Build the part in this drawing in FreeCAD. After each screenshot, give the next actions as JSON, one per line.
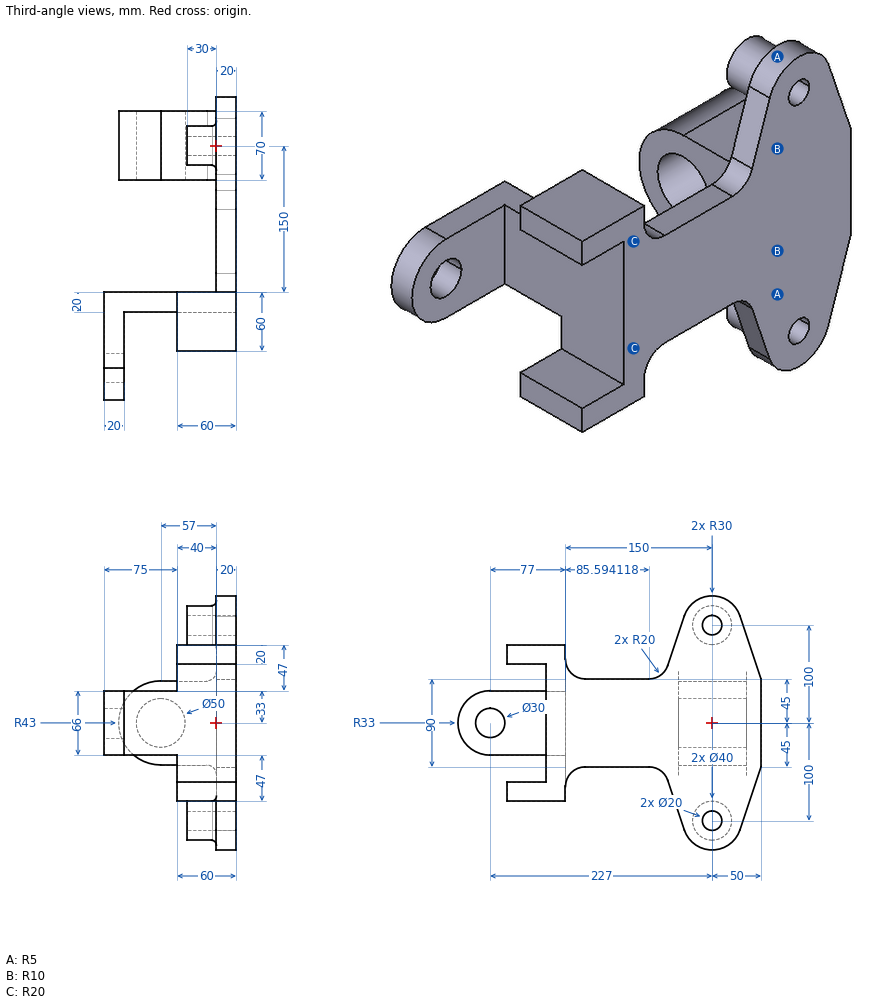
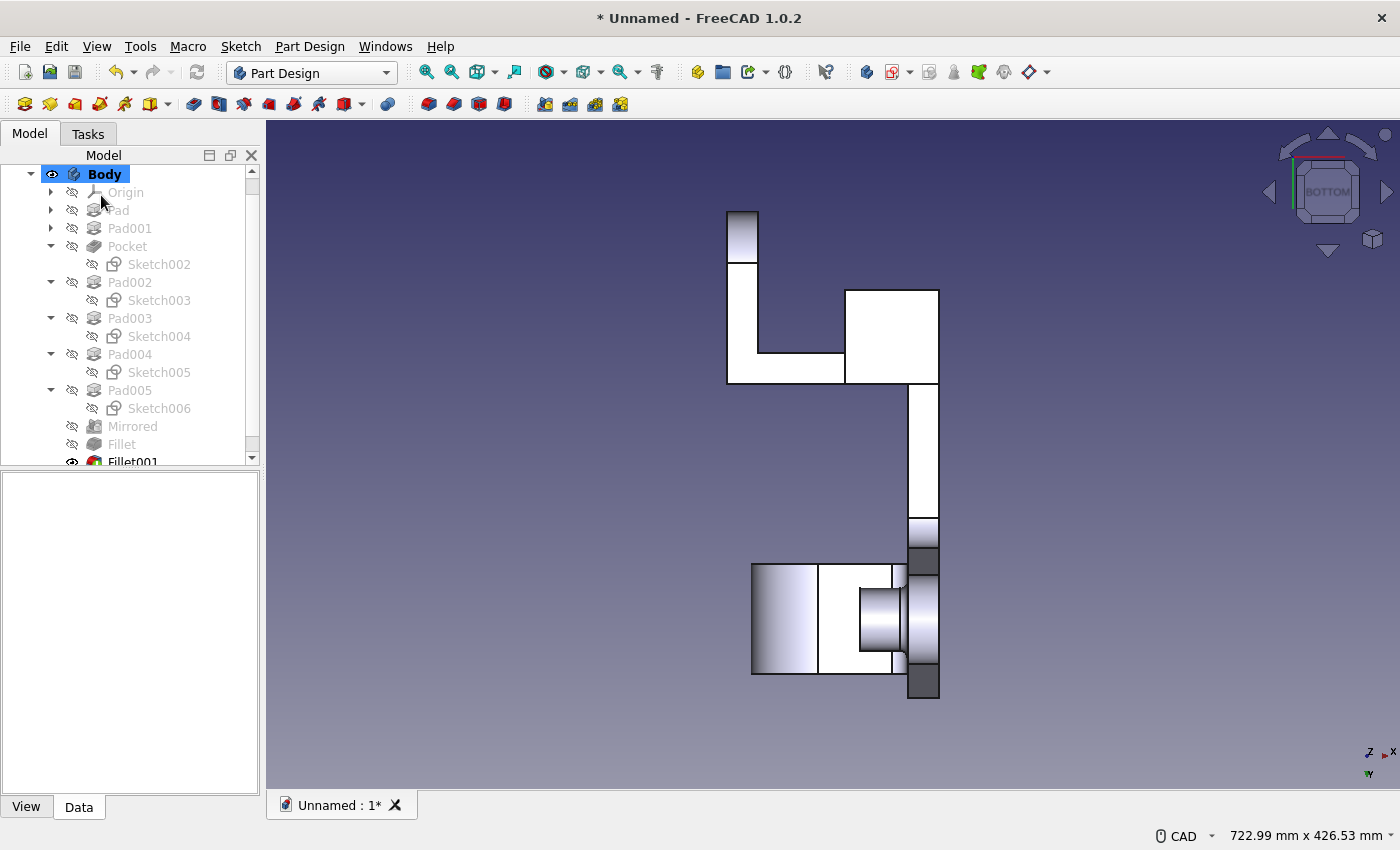
{"action": "key", "text": "4"}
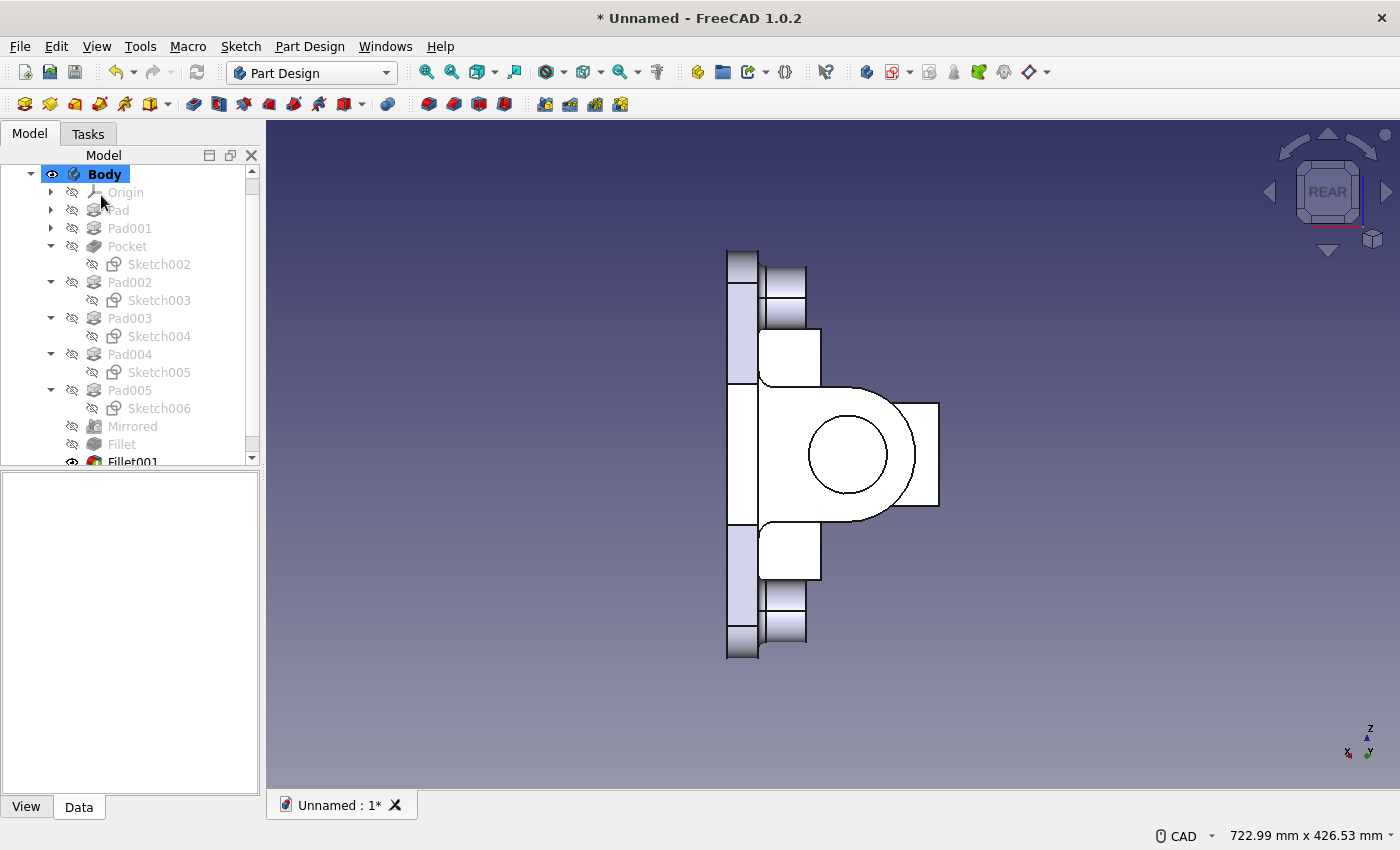
{"action": "key", "text": "6"}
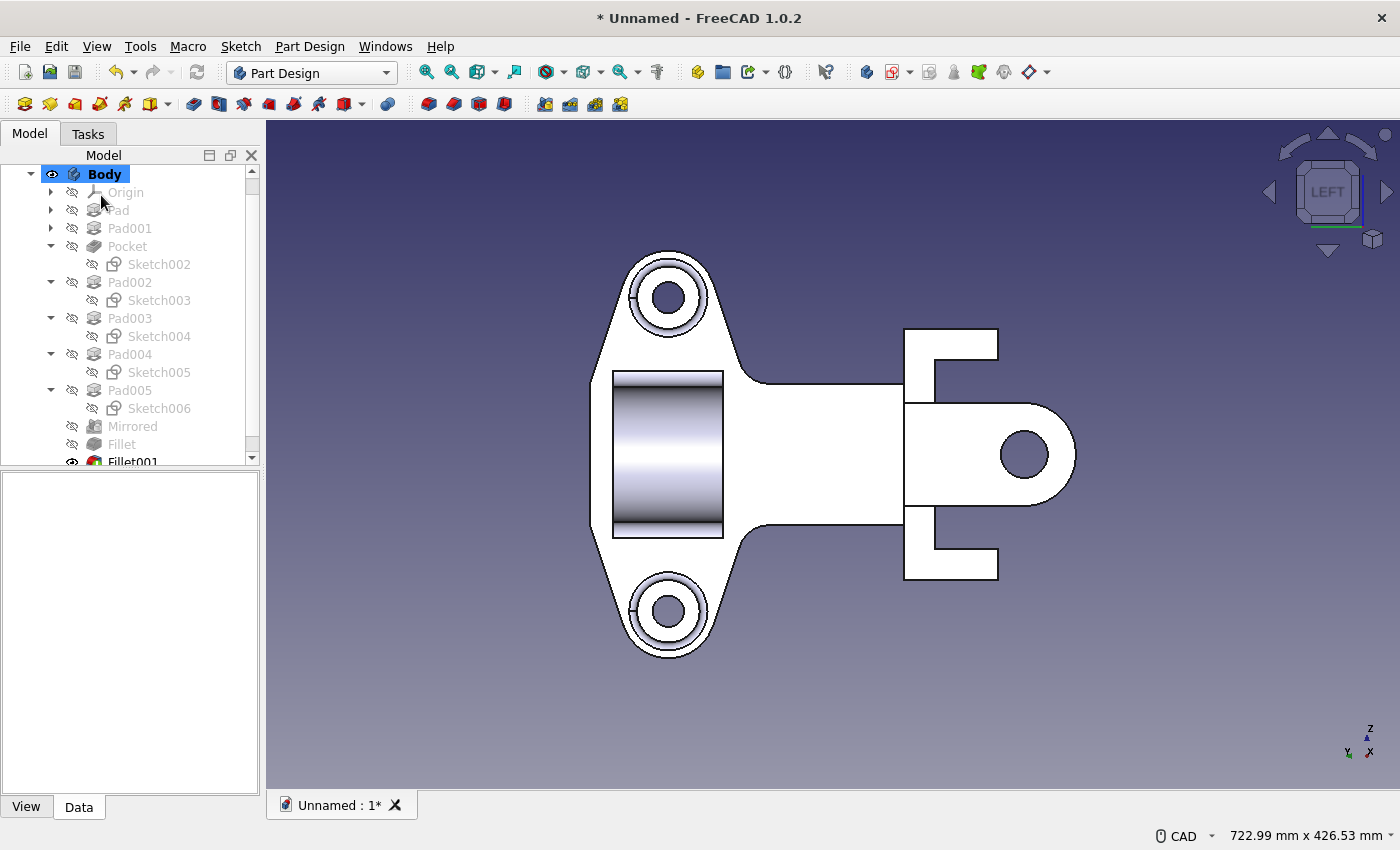
{"action": "key", "text": "v 3"}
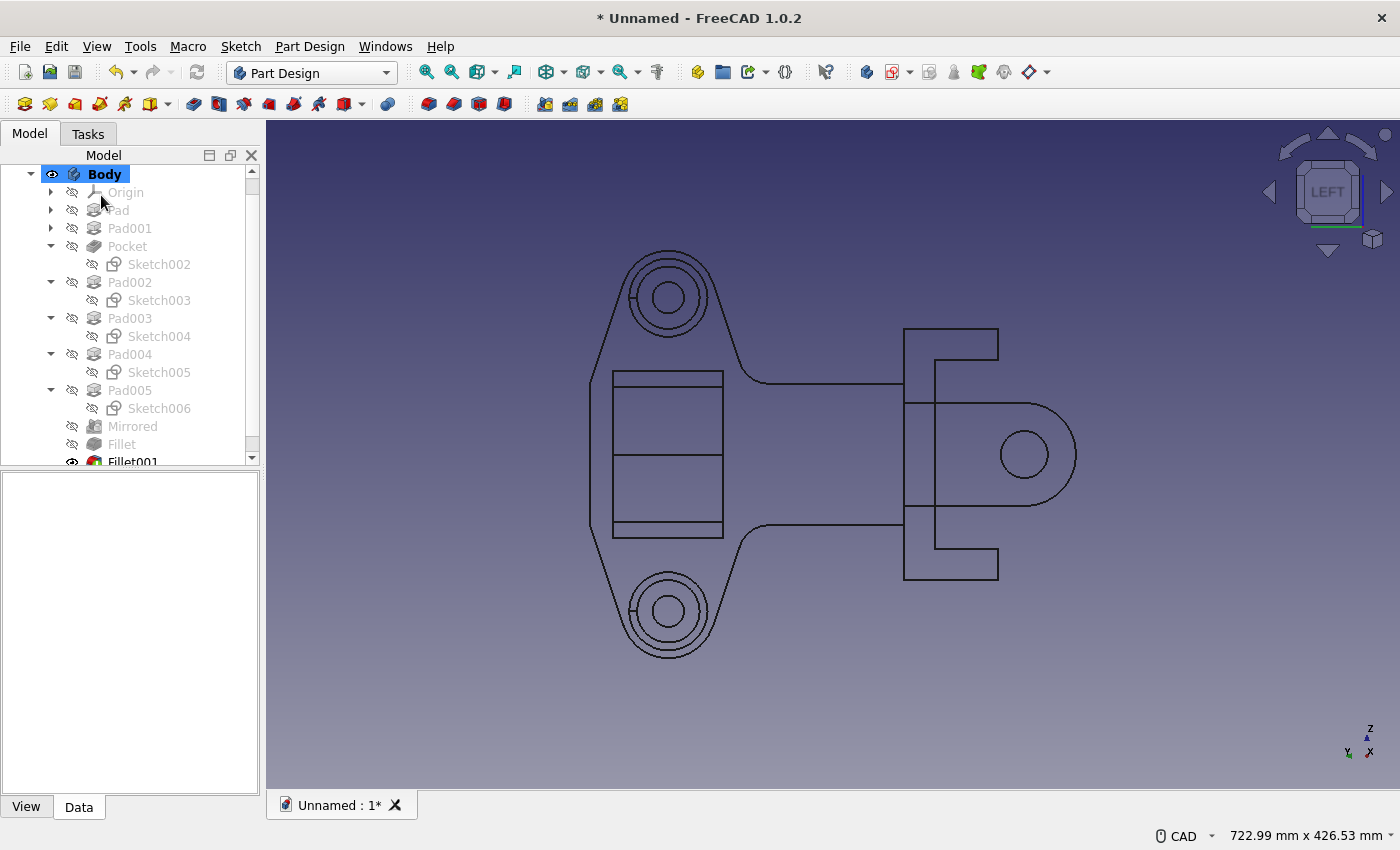
{"action": "key", "text": "0"}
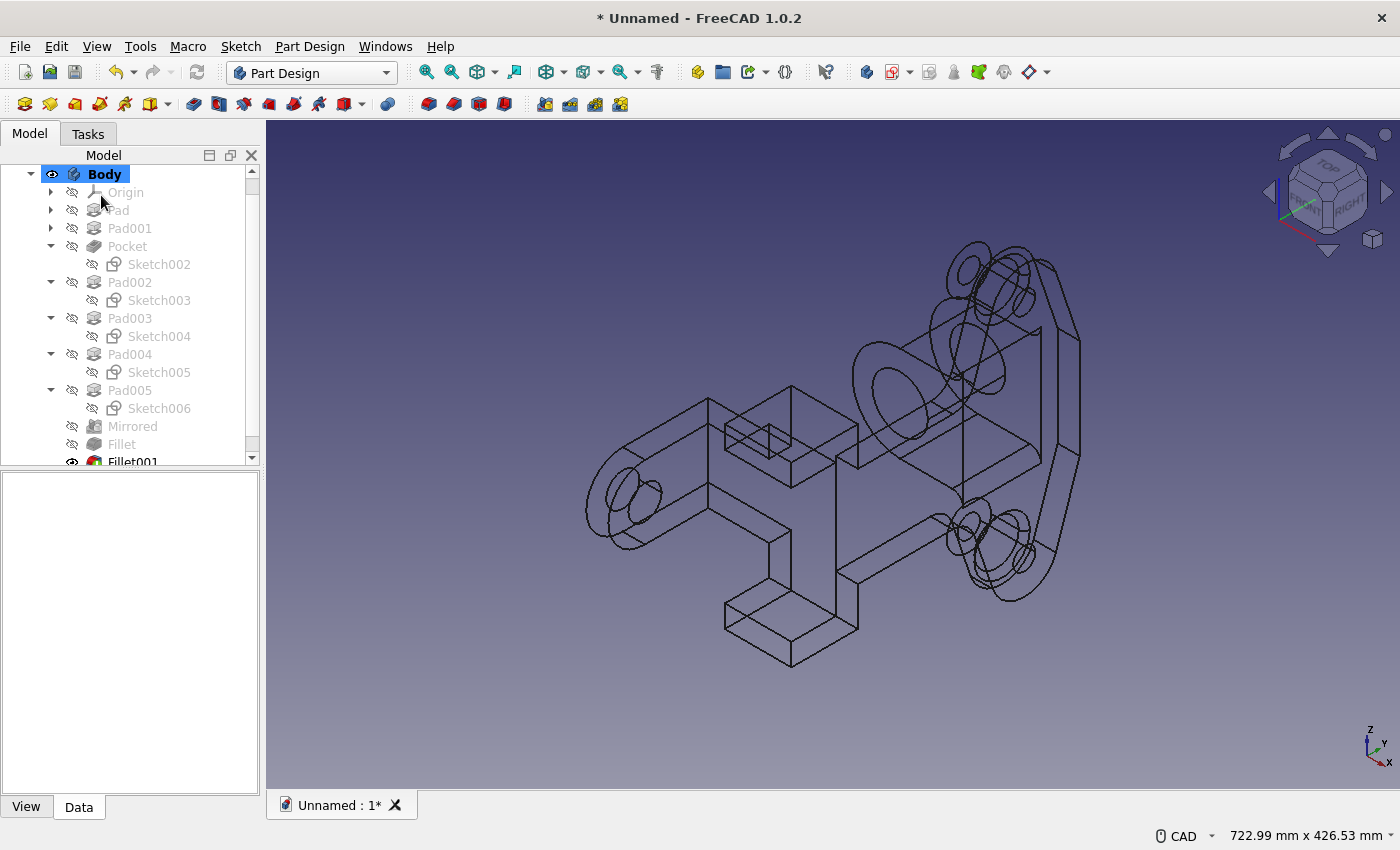
{"action": "left_click", "coordinate": [847, 577]}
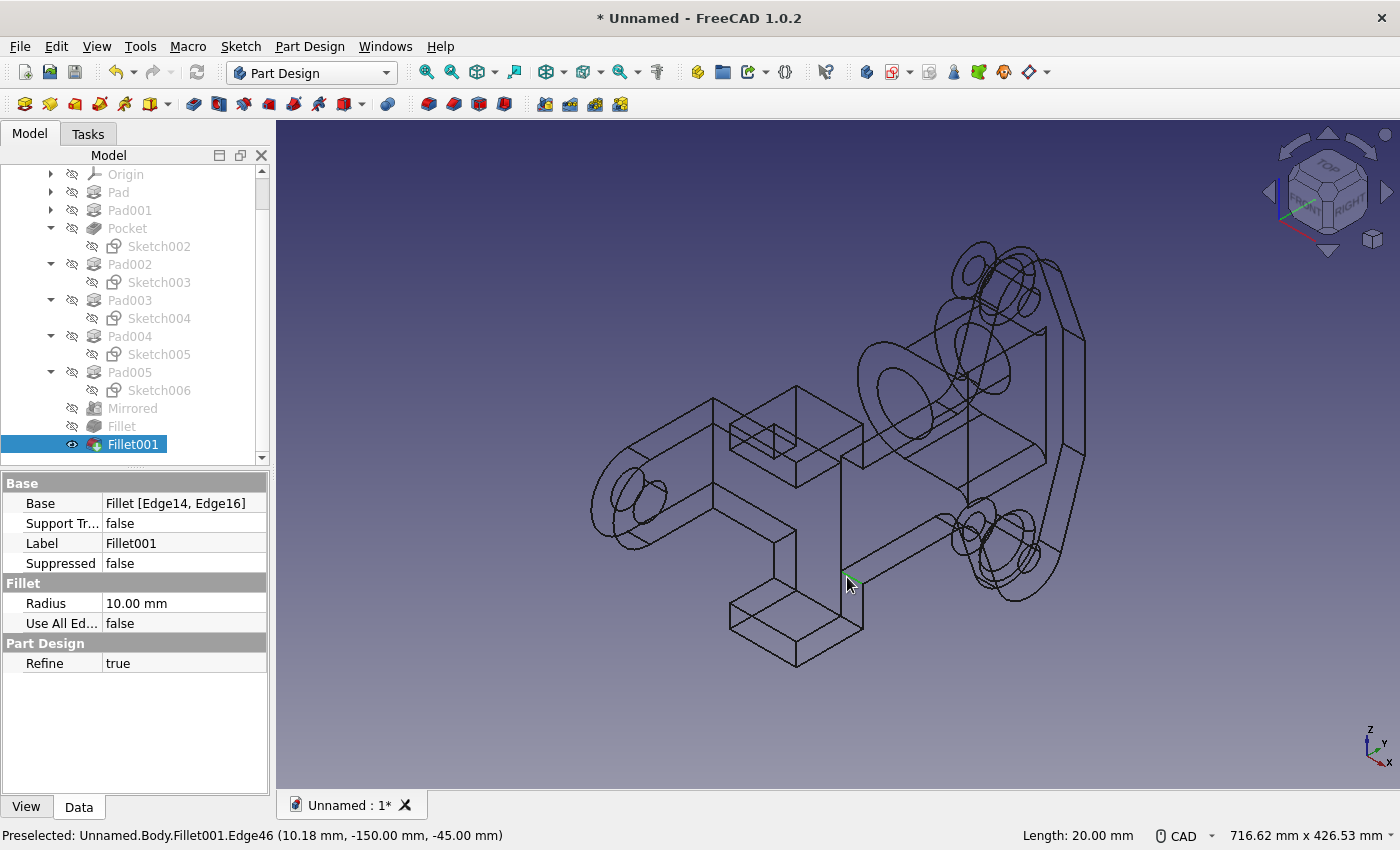
{"action": "left_click", "coordinate": [852, 462], "text": "ctrl"}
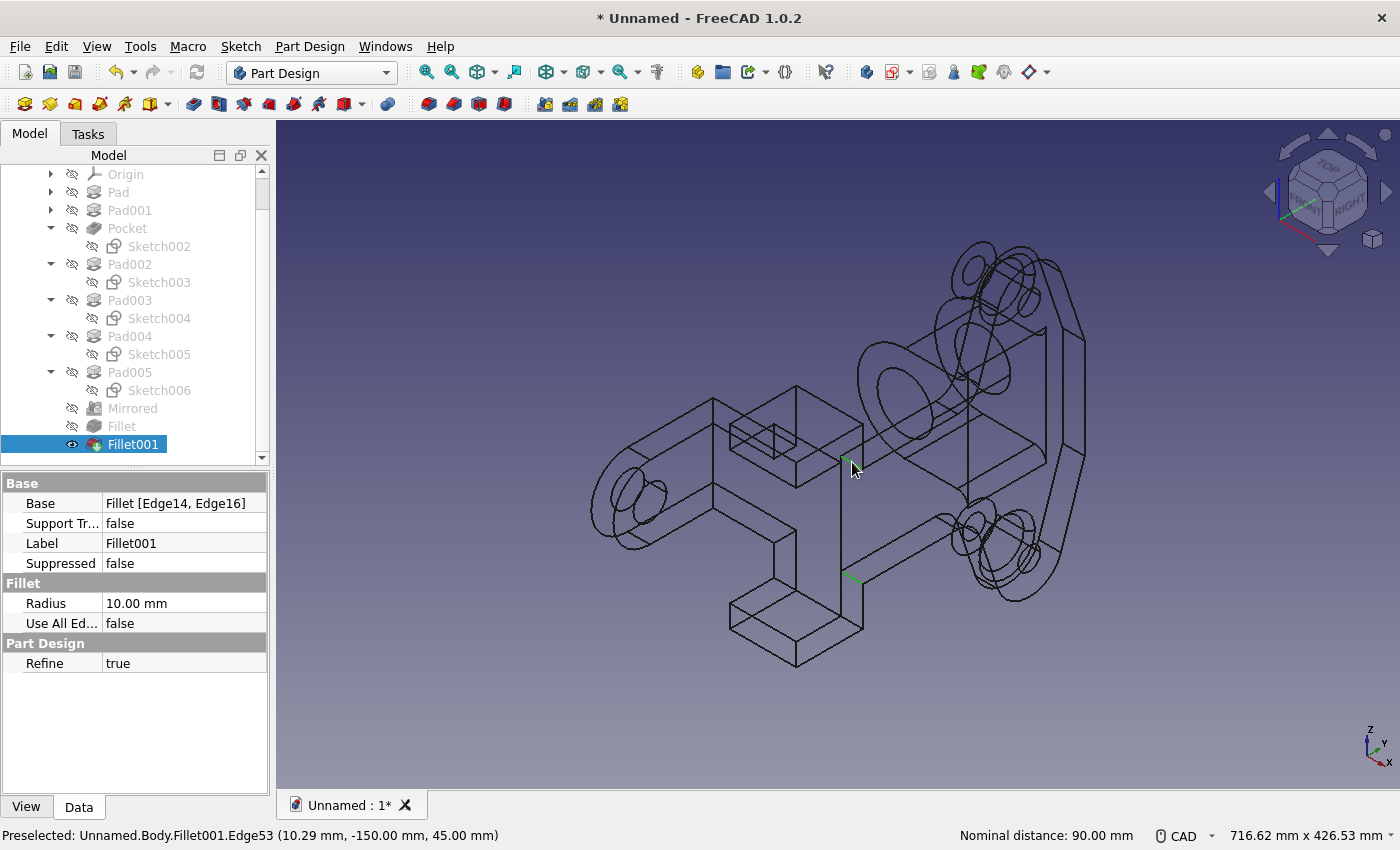
{"action": "key", "text": "v 1"}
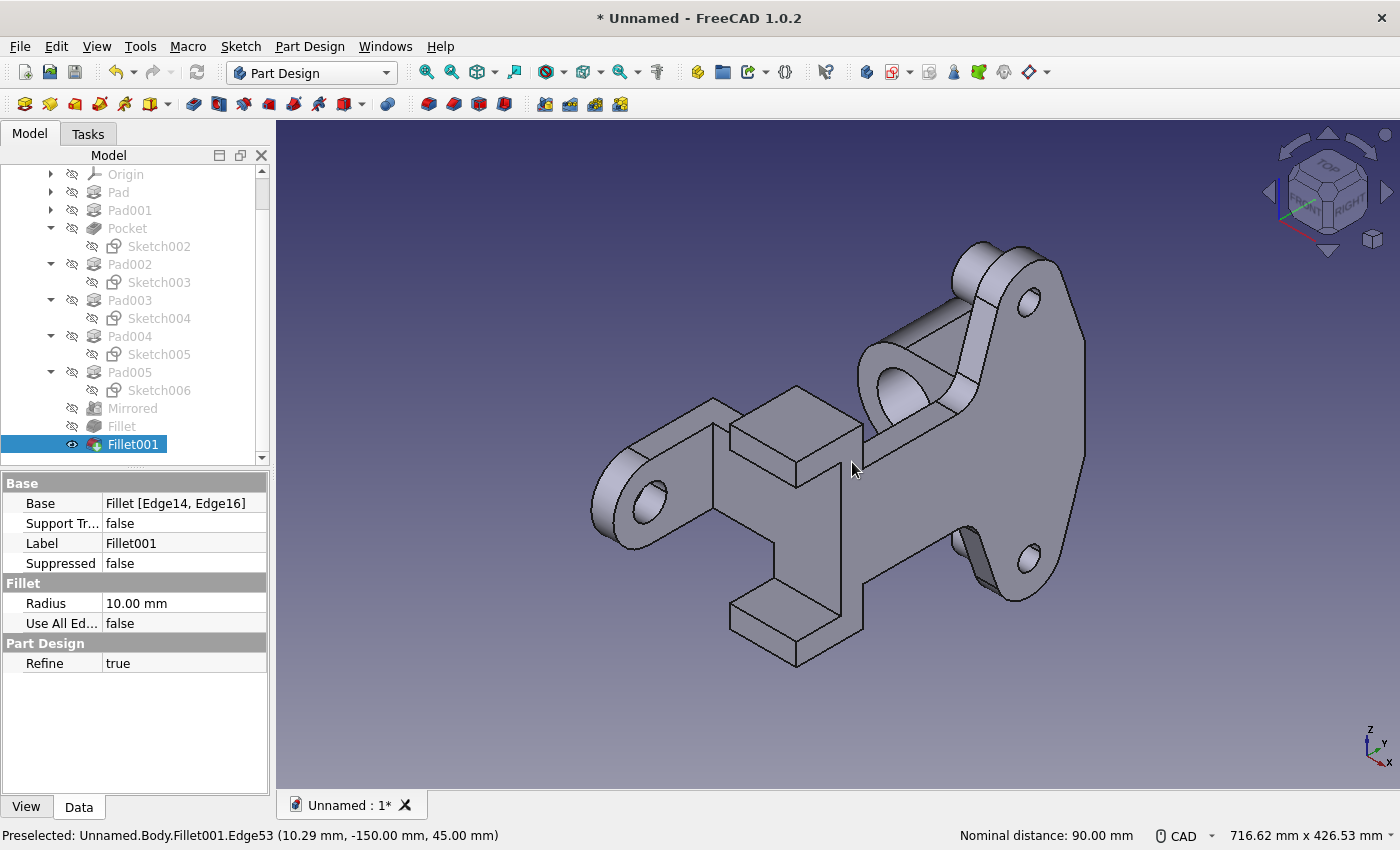
{"action": "left_click", "coordinate": [429, 104]}